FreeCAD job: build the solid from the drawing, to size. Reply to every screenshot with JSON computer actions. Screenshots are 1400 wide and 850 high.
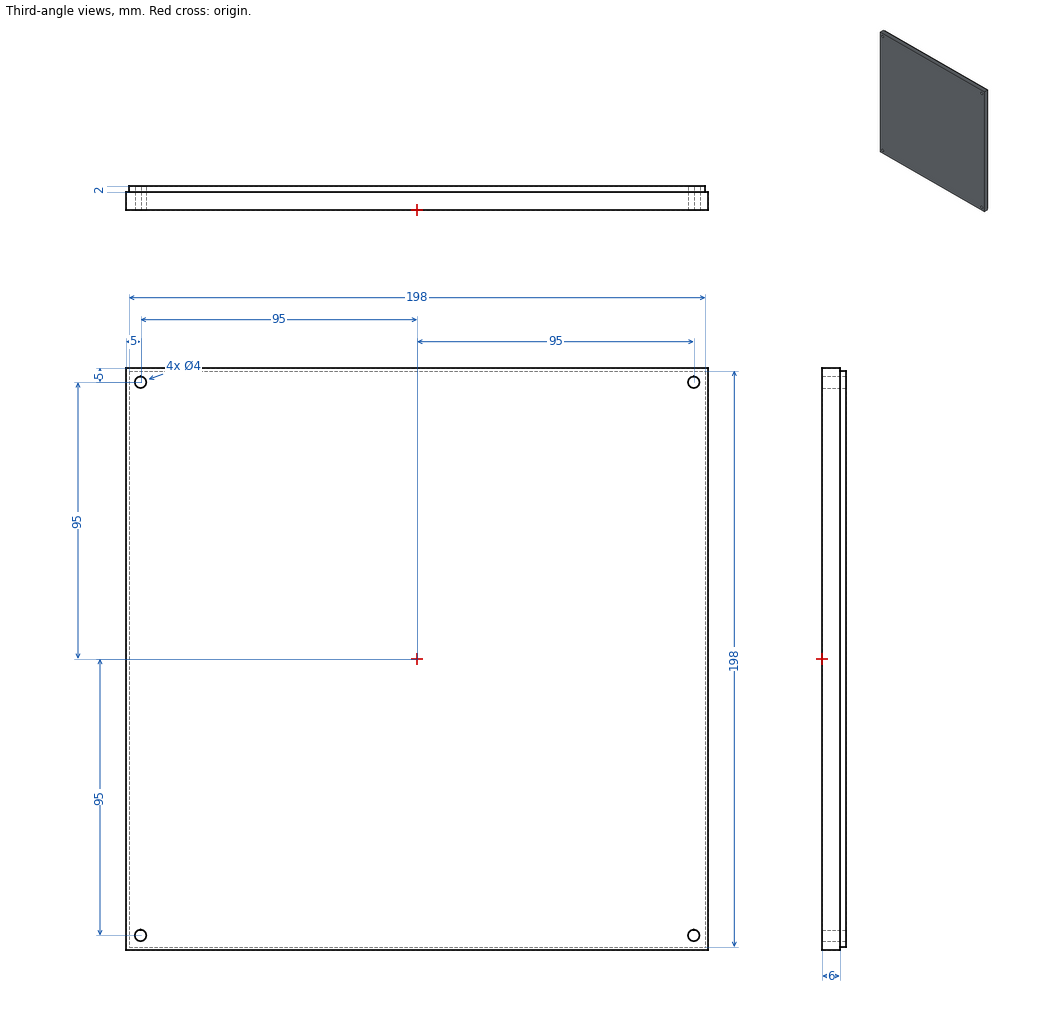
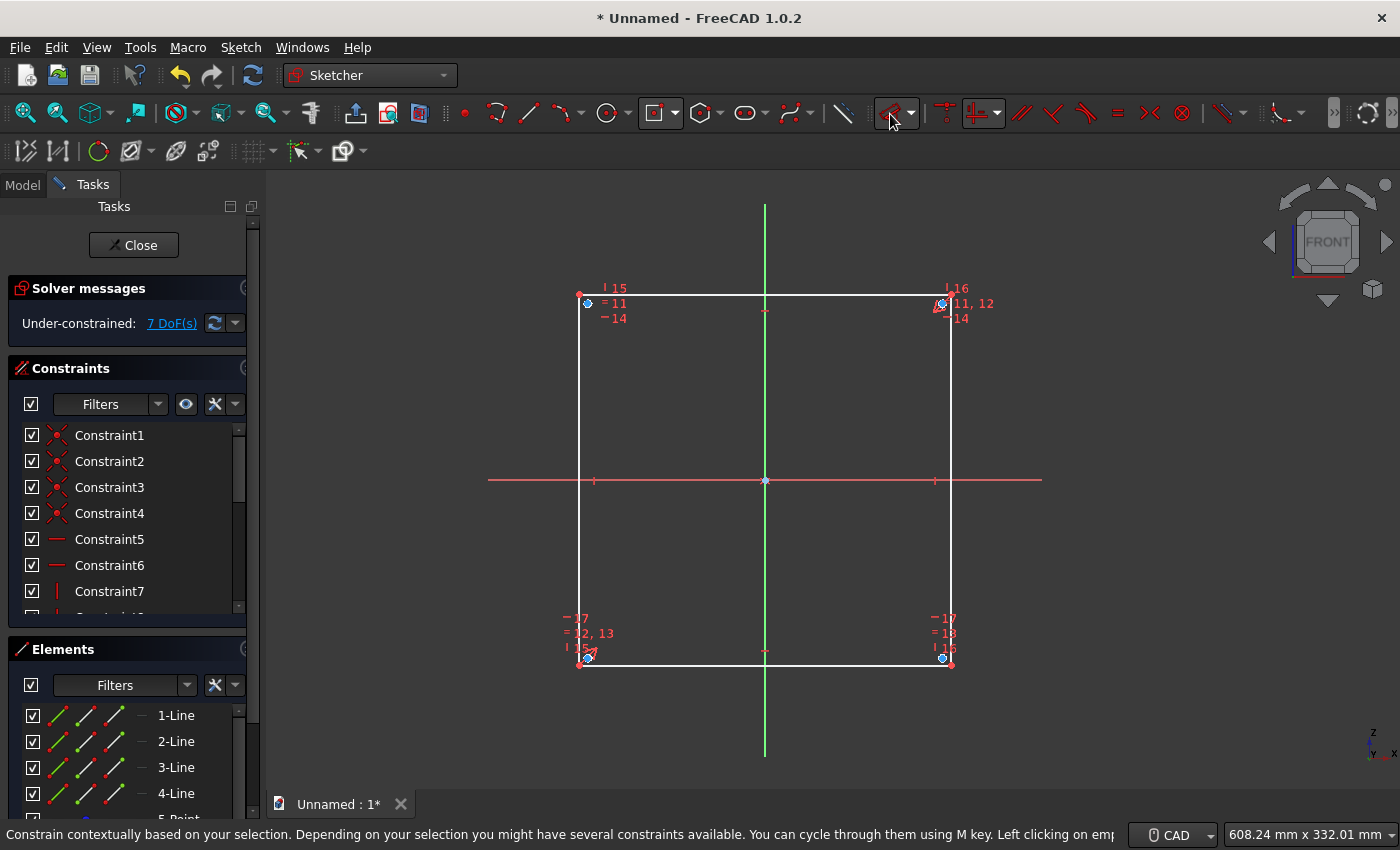
{"action": "scroll", "coordinate": [588, 307], "scroll_direction": "up", "scroll_amount": 9}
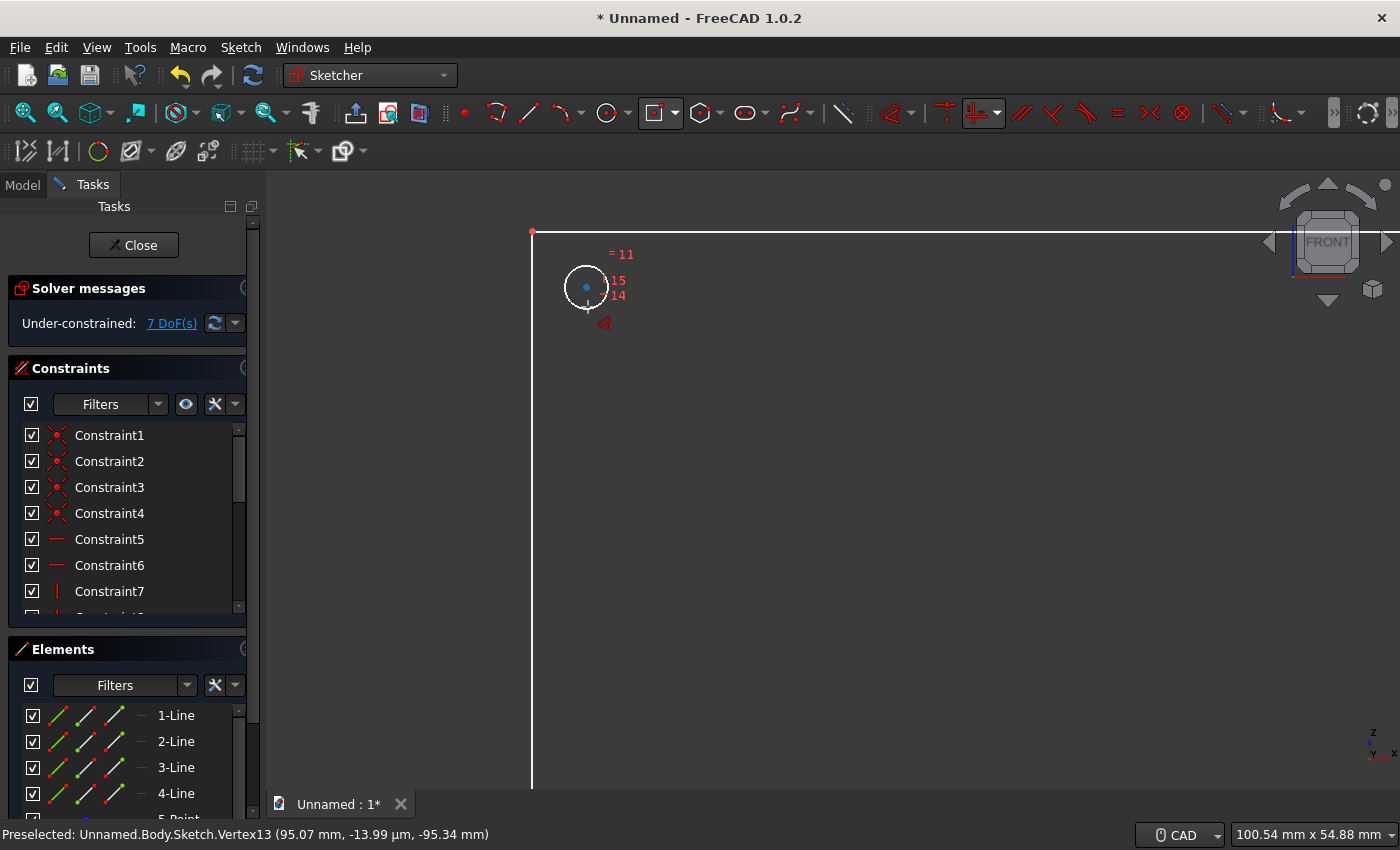
{"action": "left_click", "coordinate": [586, 309]}
{"action": "left_click", "coordinate": [585, 341]}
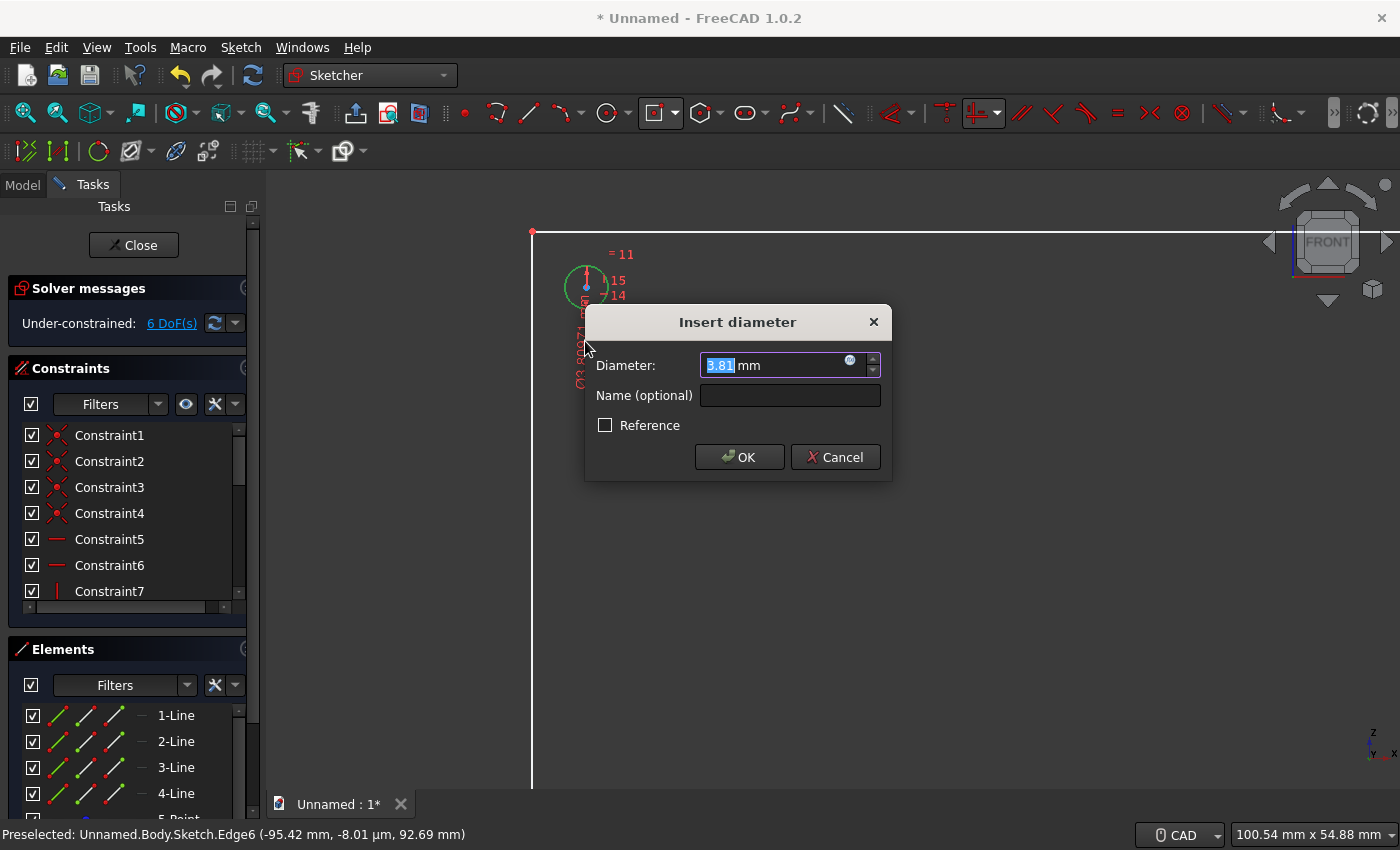
{"action": "type", "text": "4"}
{"action": "key", "text": "Return"}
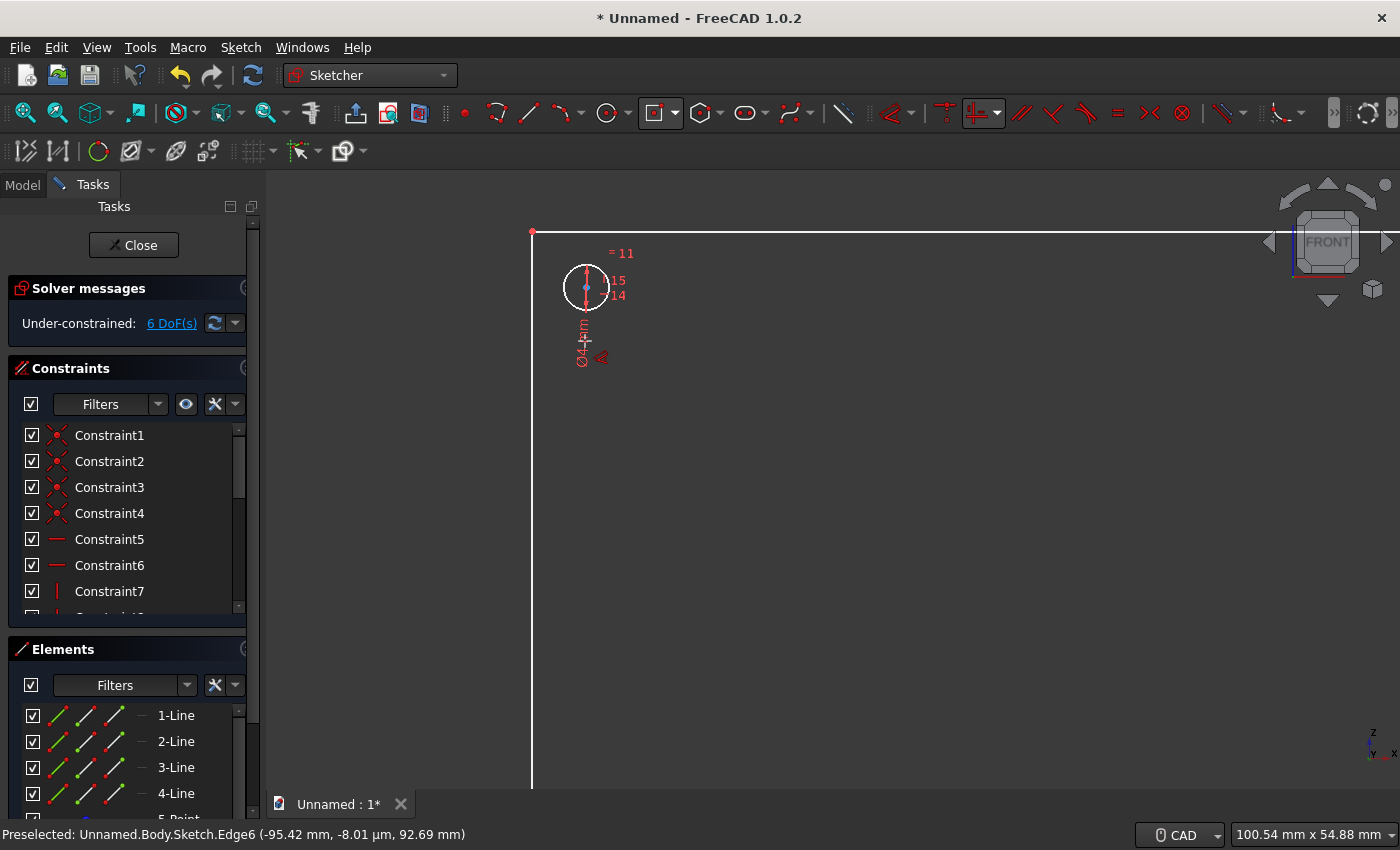
{"action": "scroll", "coordinate": [587, 306], "scroll_direction": "down", "scroll_amount": 9}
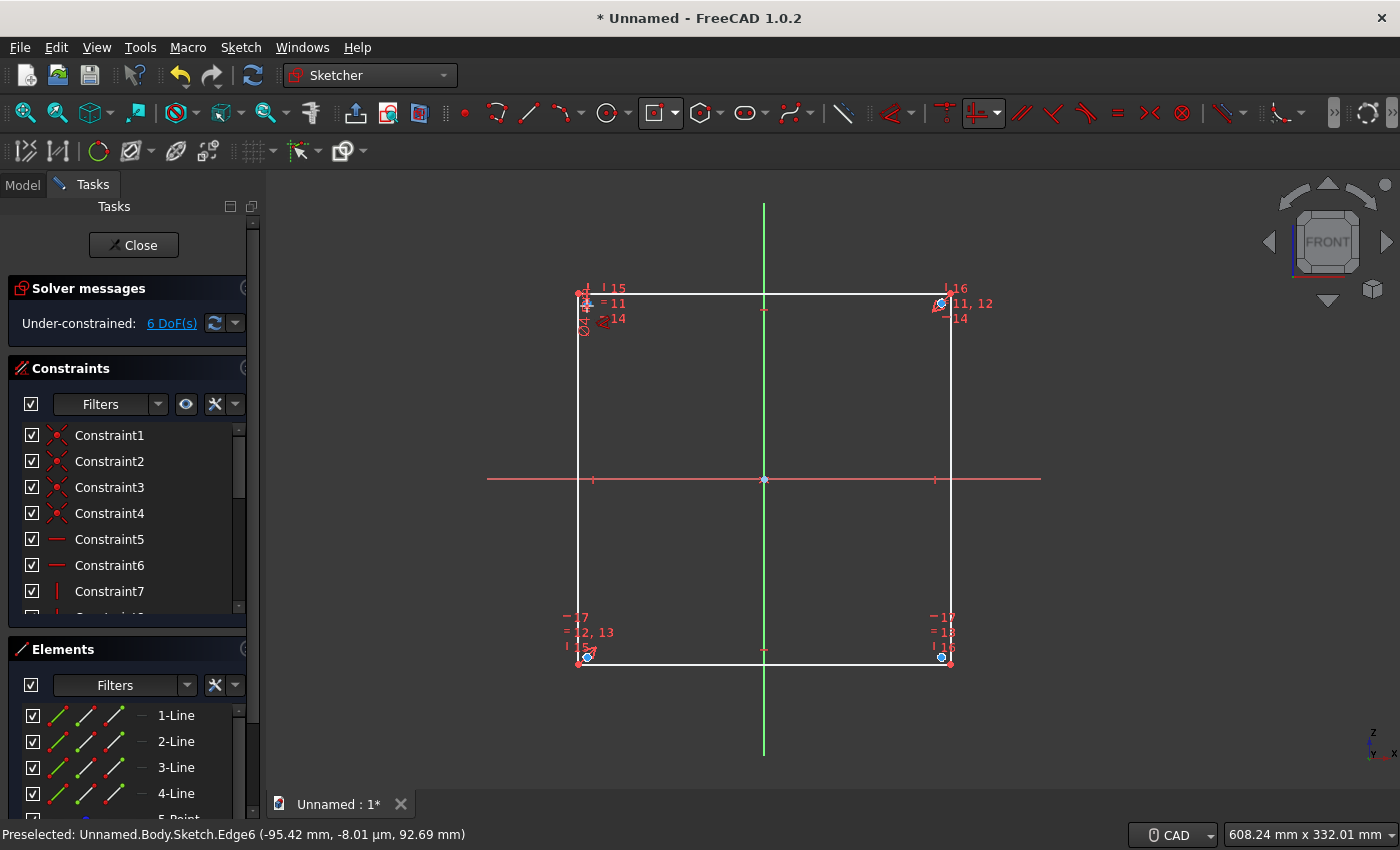
{"action": "left_click", "coordinate": [587, 303]}
{"action": "left_click", "coordinate": [676, 269]}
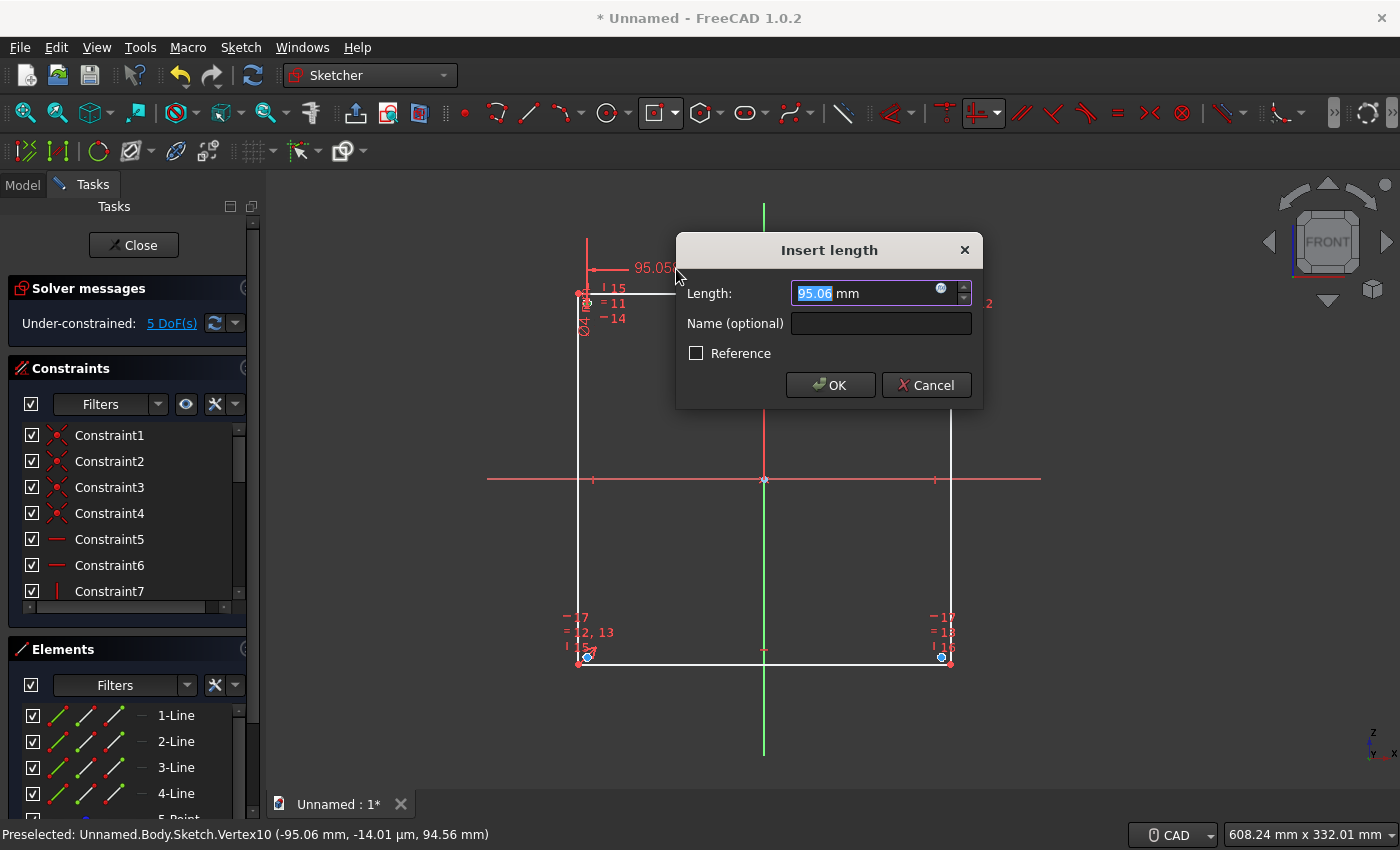
{"action": "type", "text": "95"}
{"action": "key", "text": "Return"}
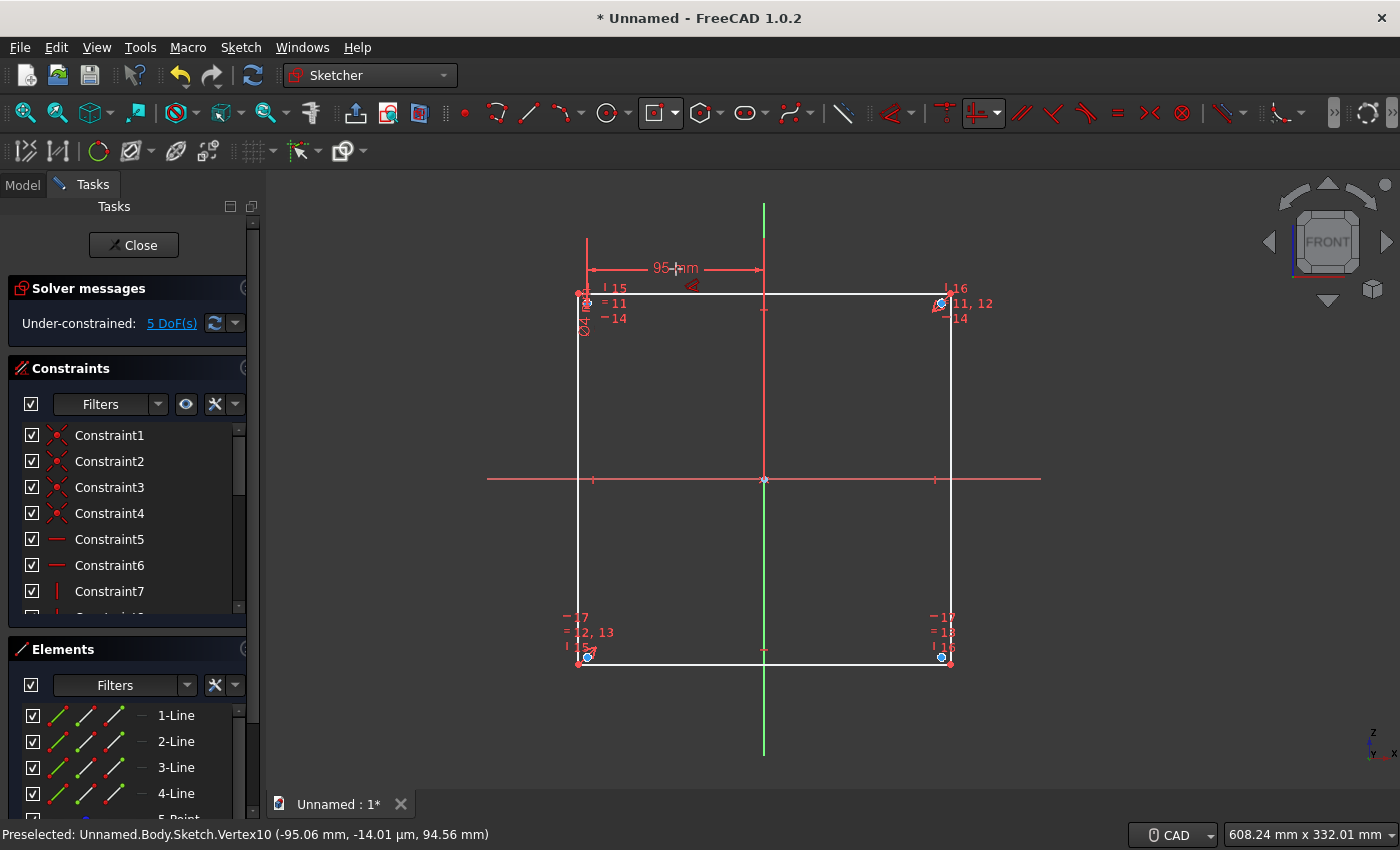
{"action": "left_click", "coordinate": [587, 303]}
{"action": "left_click", "coordinate": [553, 391]}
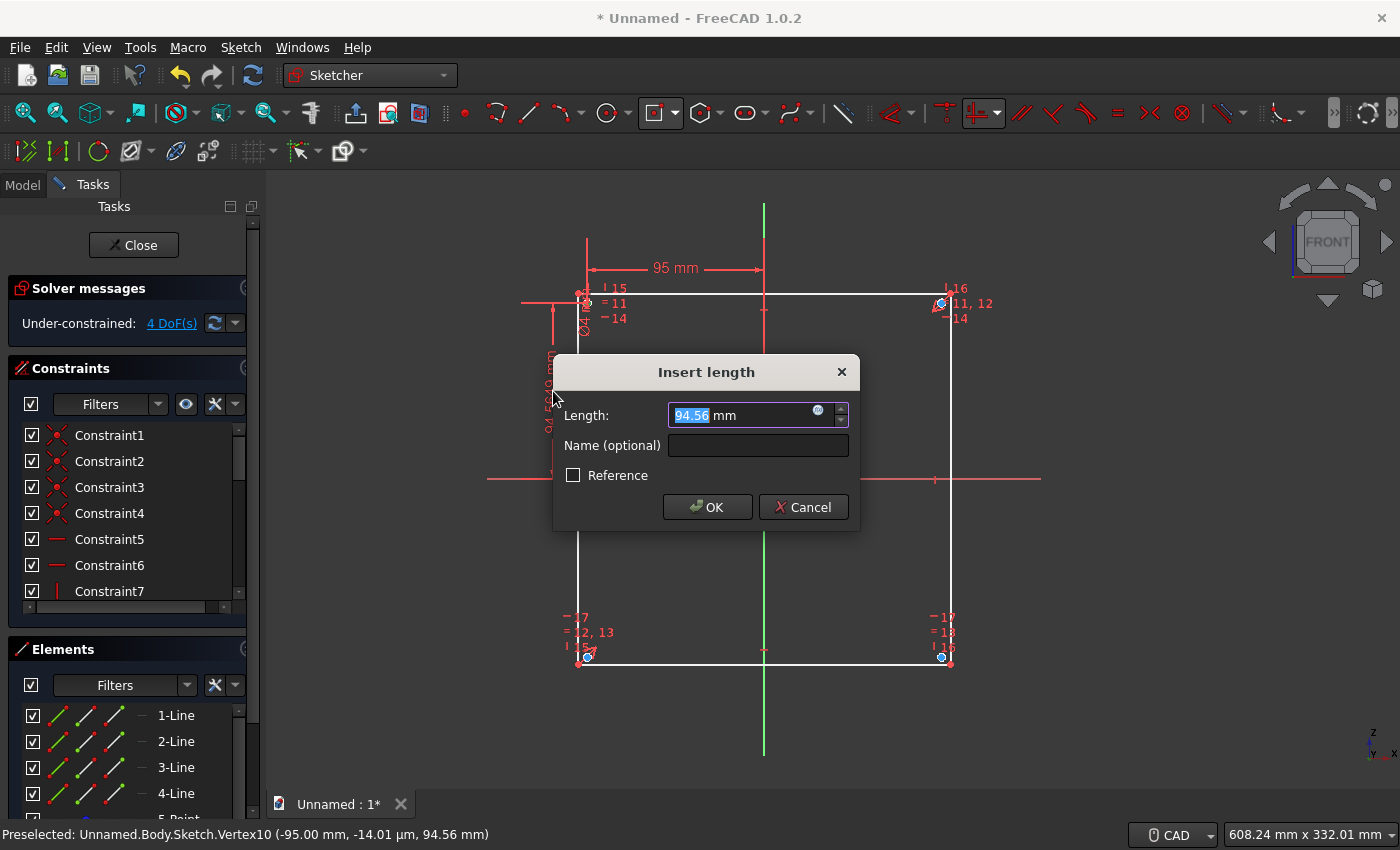
{"action": "type", "text": "95"}
{"action": "key", "text": "Return"}